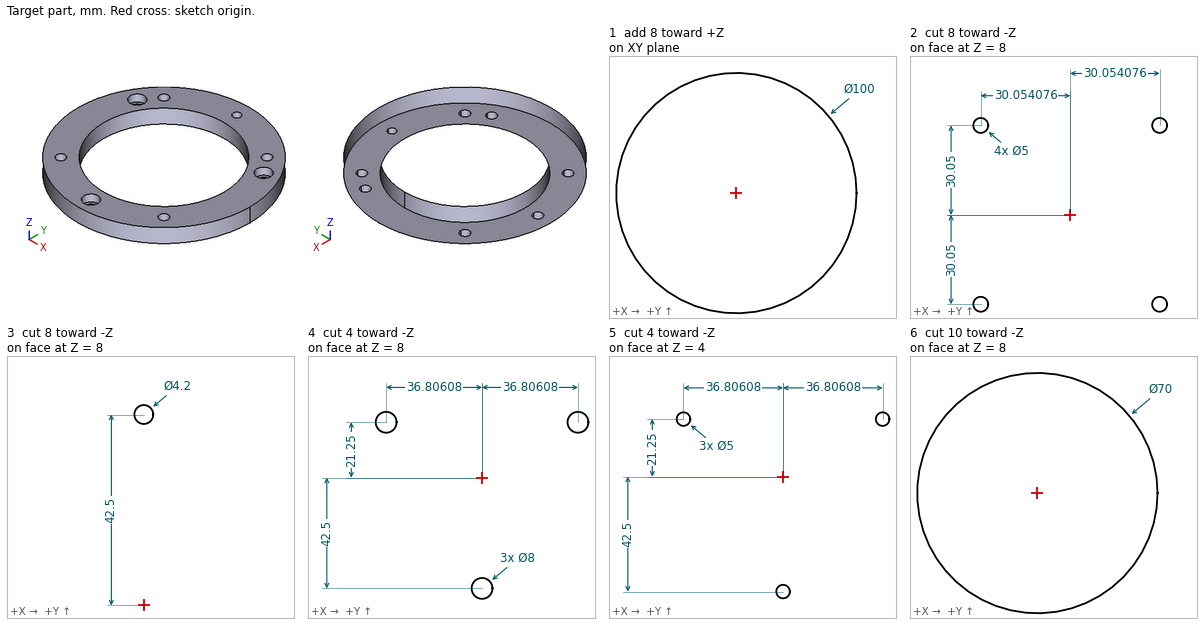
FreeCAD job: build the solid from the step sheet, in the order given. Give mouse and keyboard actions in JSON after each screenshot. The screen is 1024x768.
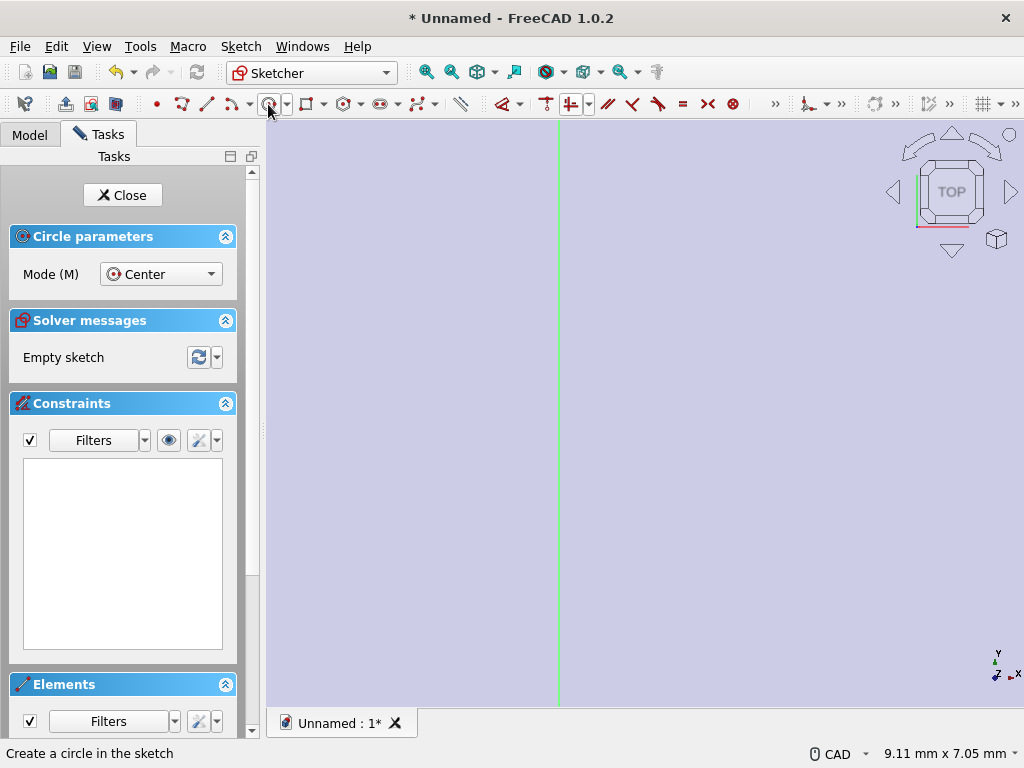
{"action": "left_click", "coordinate": [559, 413]}
{"action": "mouse_move", "coordinate": [683, 289]}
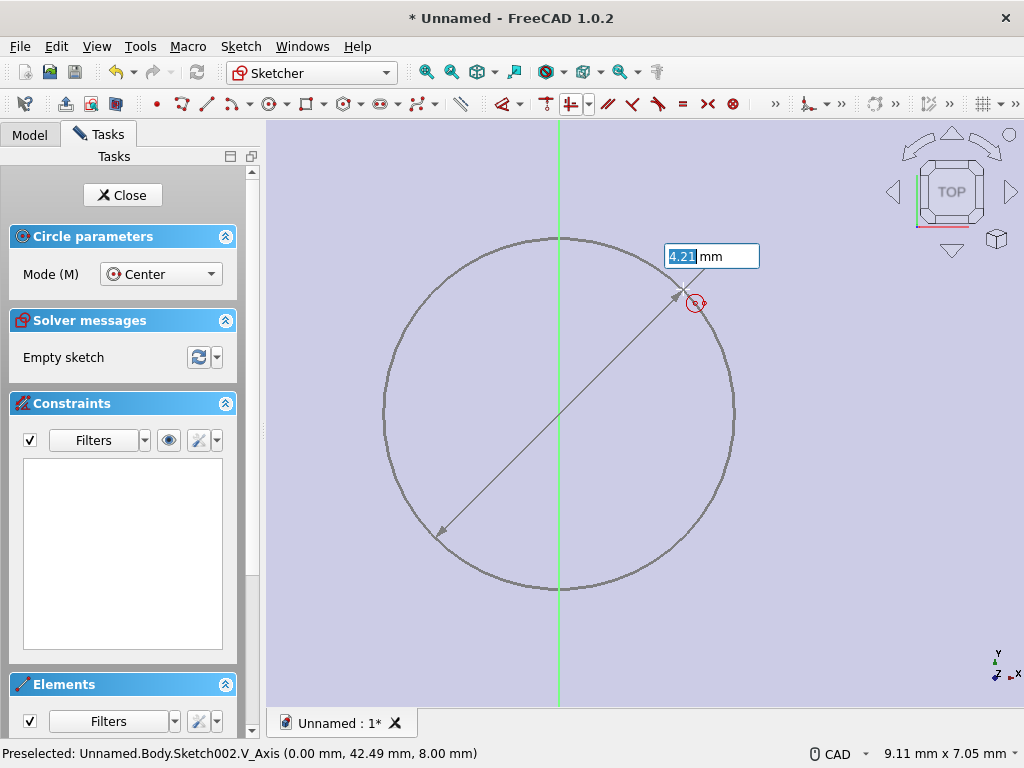
{"action": "type", "text": "4.2"}
{"action": "key", "text": "Return"}
{"action": "key", "text": "Escape"}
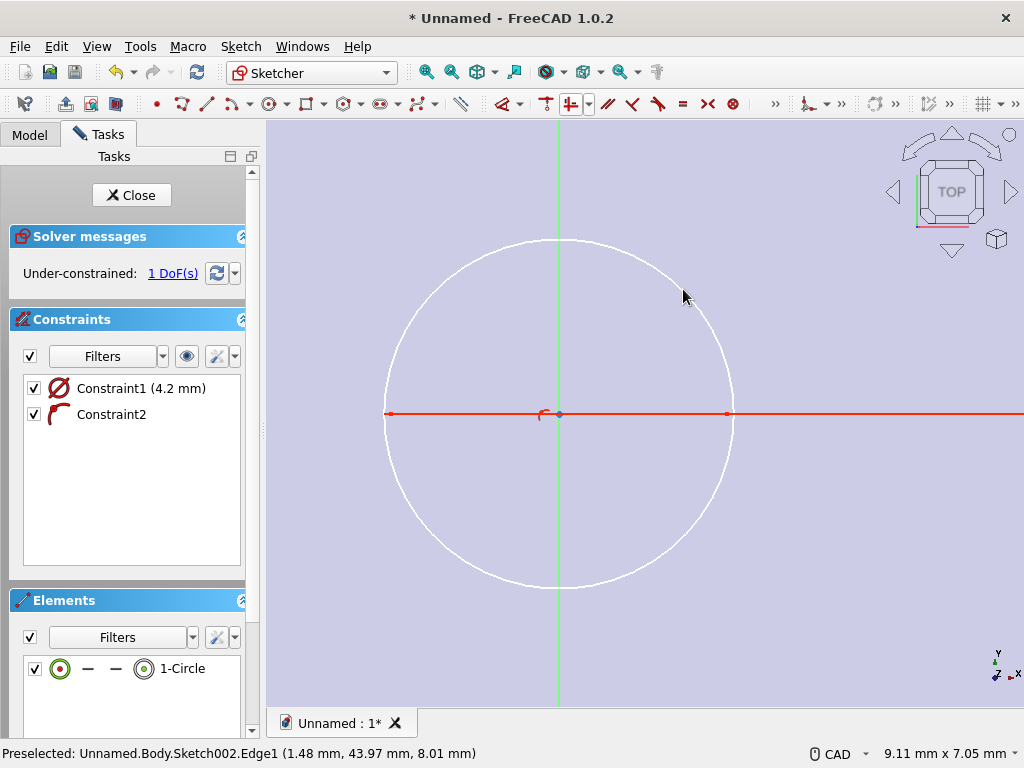
{"action": "key", "text": "d"}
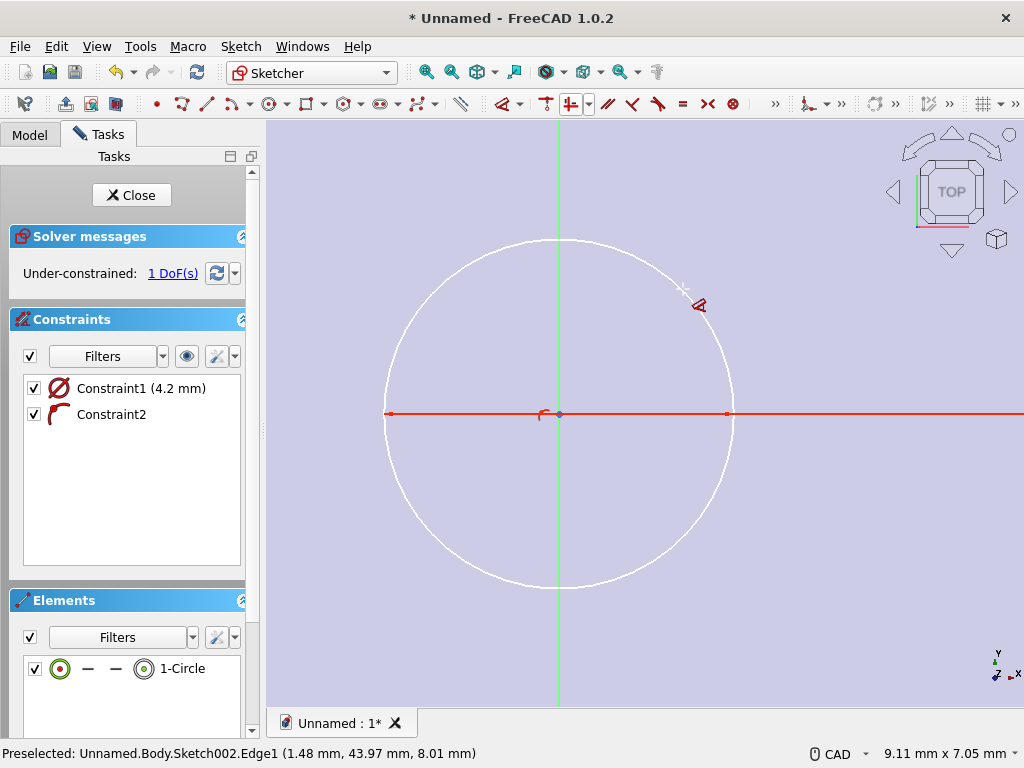
{"action": "left_click", "coordinate": [559, 414]}
{"action": "left_click", "coordinate": [593, 547]}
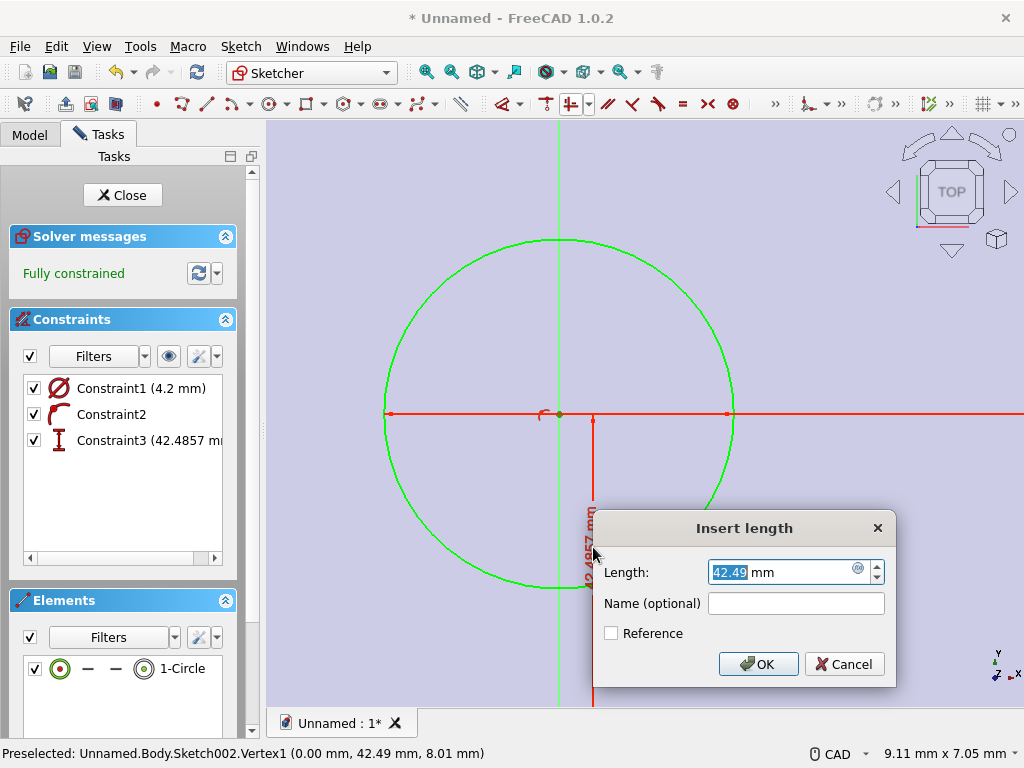
{"action": "type", "text": "42.5"}
{"action": "key", "text": "Return"}
{"action": "key", "text": "Escape"}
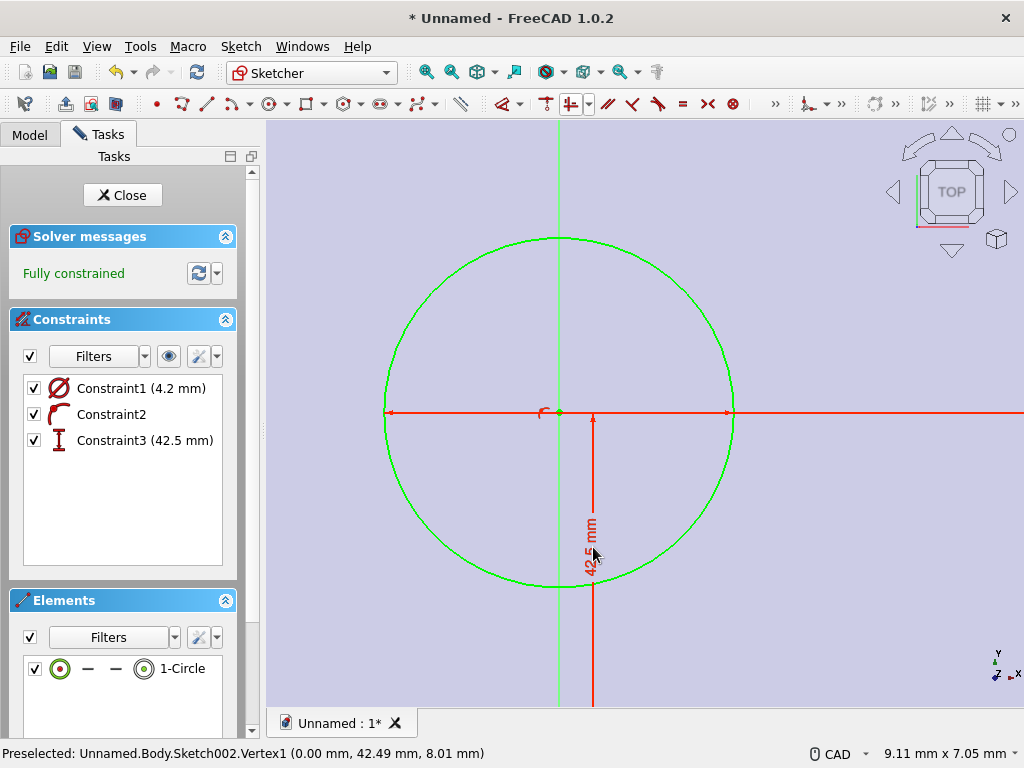
{"action": "left_click", "coordinate": [123, 195]}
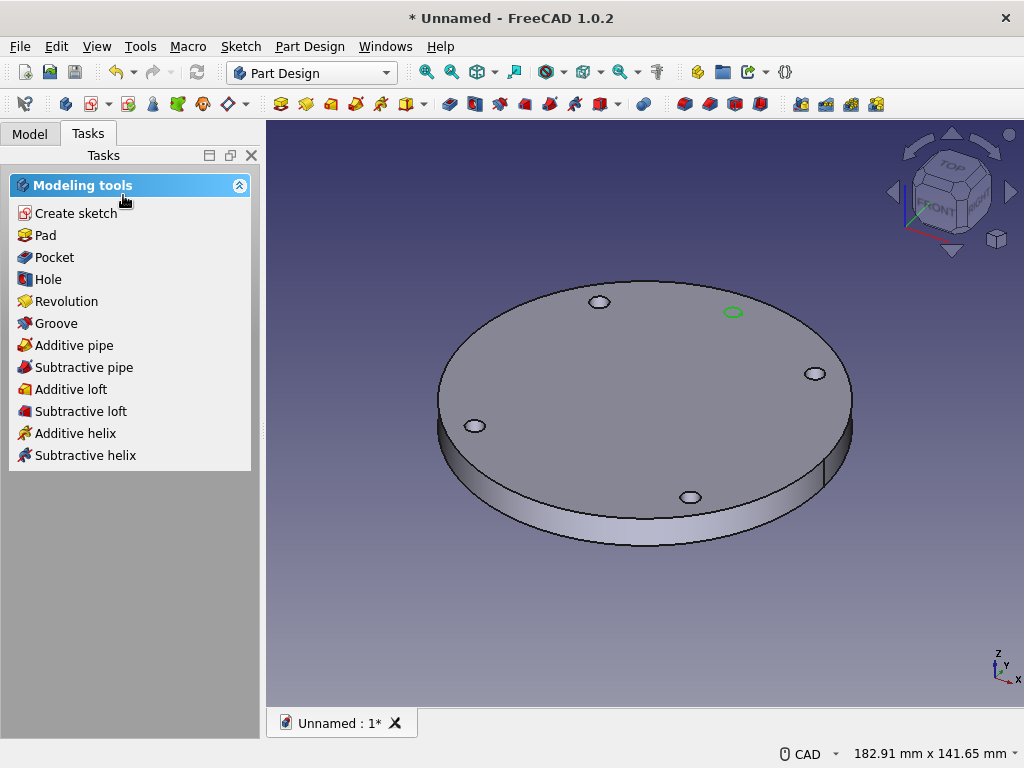
{"action": "left_click", "coordinate": [450, 104]}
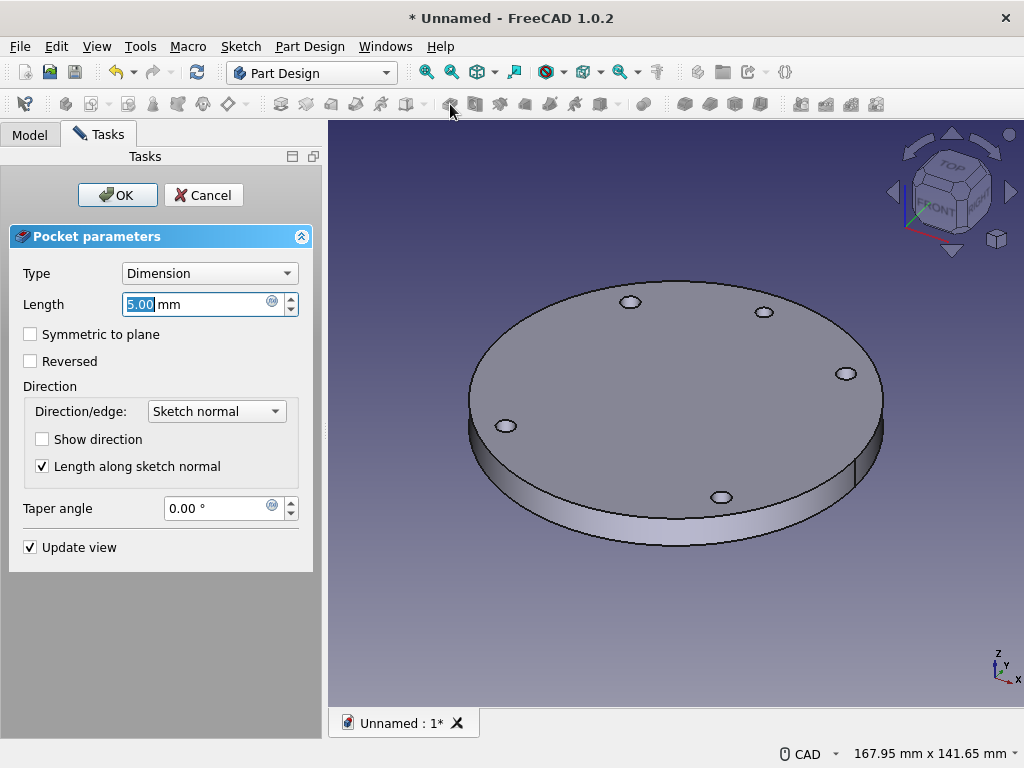
{"action": "type", "text": "8"}
{"action": "key", "text": "Tab"}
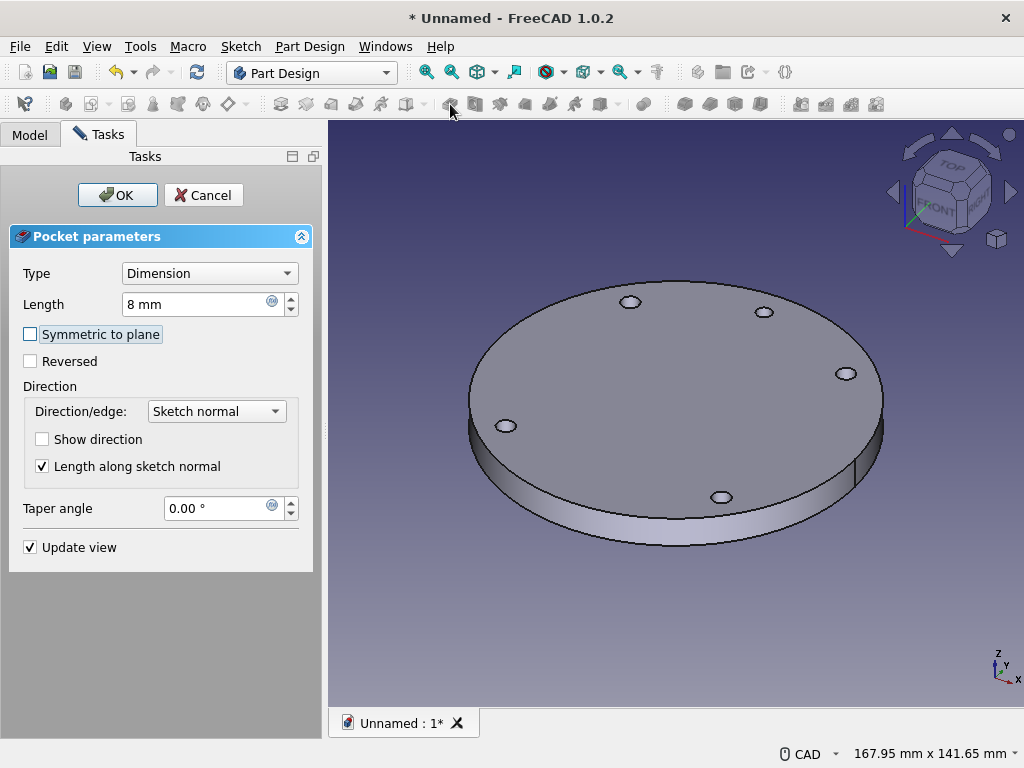
{"action": "left_click", "coordinate": [118, 195]}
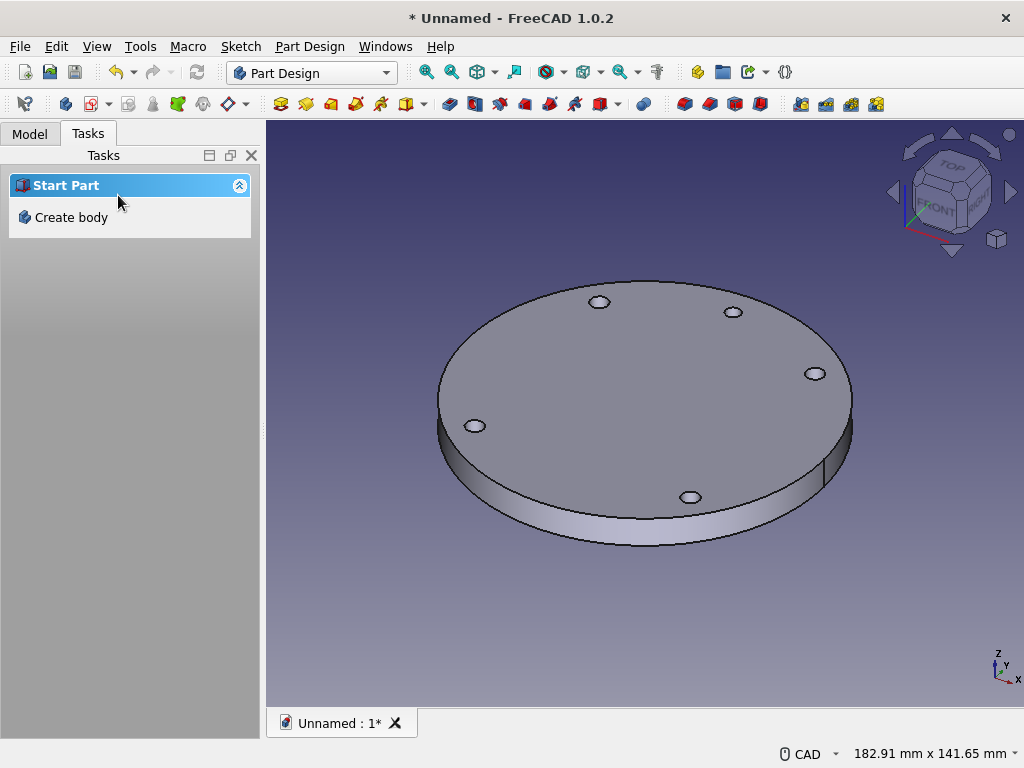
{"action": "left_click", "coordinate": [645, 399]}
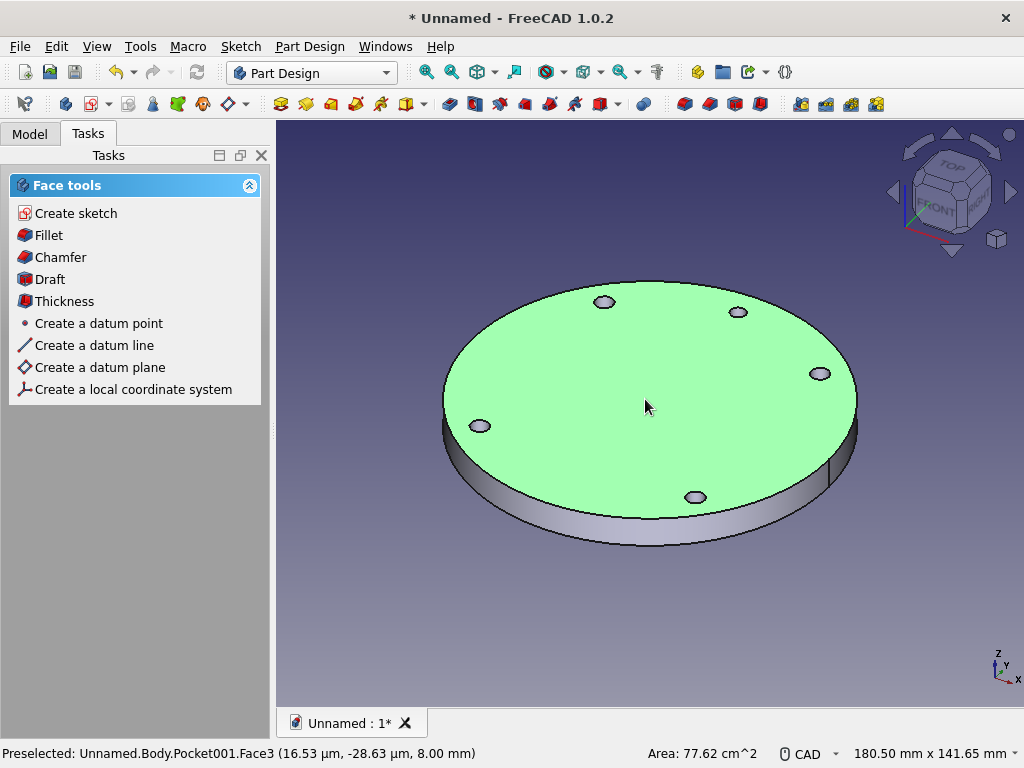
{"action": "left_click", "coordinate": [90, 104]}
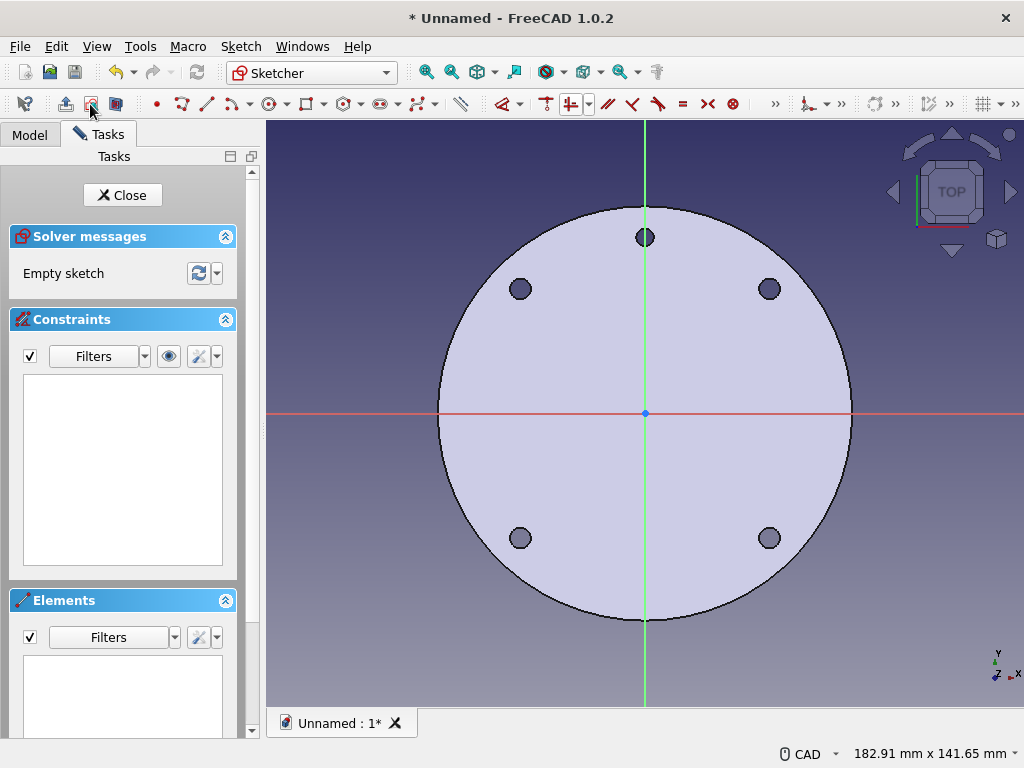
{"action": "left_click", "coordinate": [268, 104]}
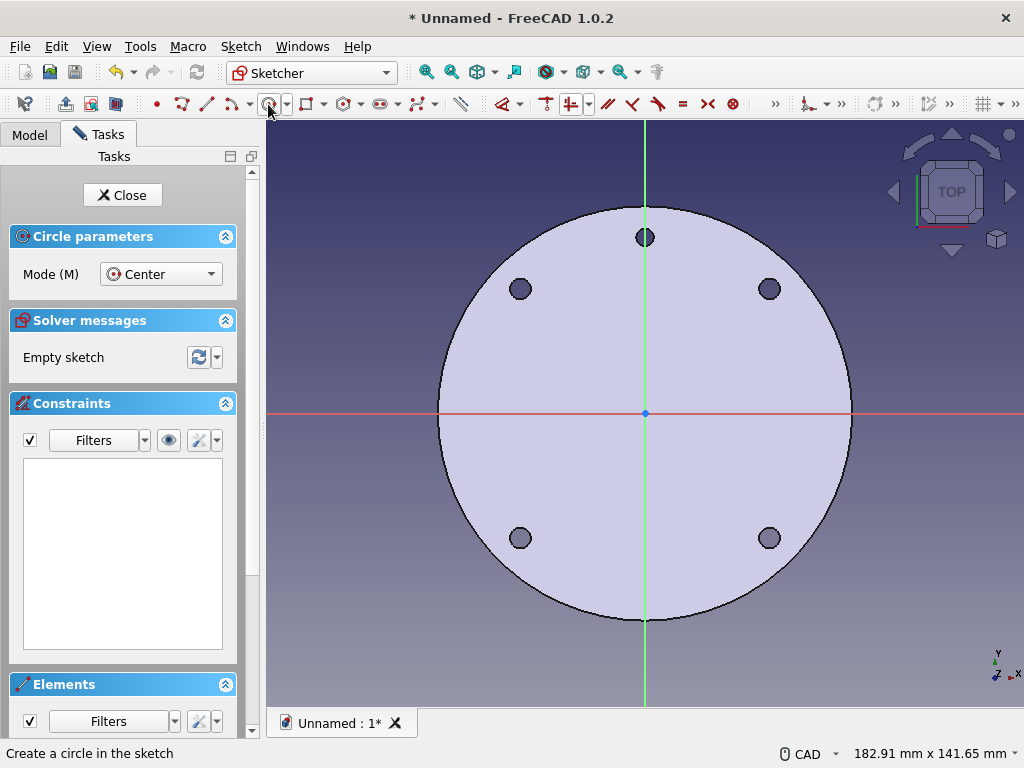
{"action": "scroll", "coordinate": [645, 590], "scroll_direction": "up", "scroll_amount": 2}